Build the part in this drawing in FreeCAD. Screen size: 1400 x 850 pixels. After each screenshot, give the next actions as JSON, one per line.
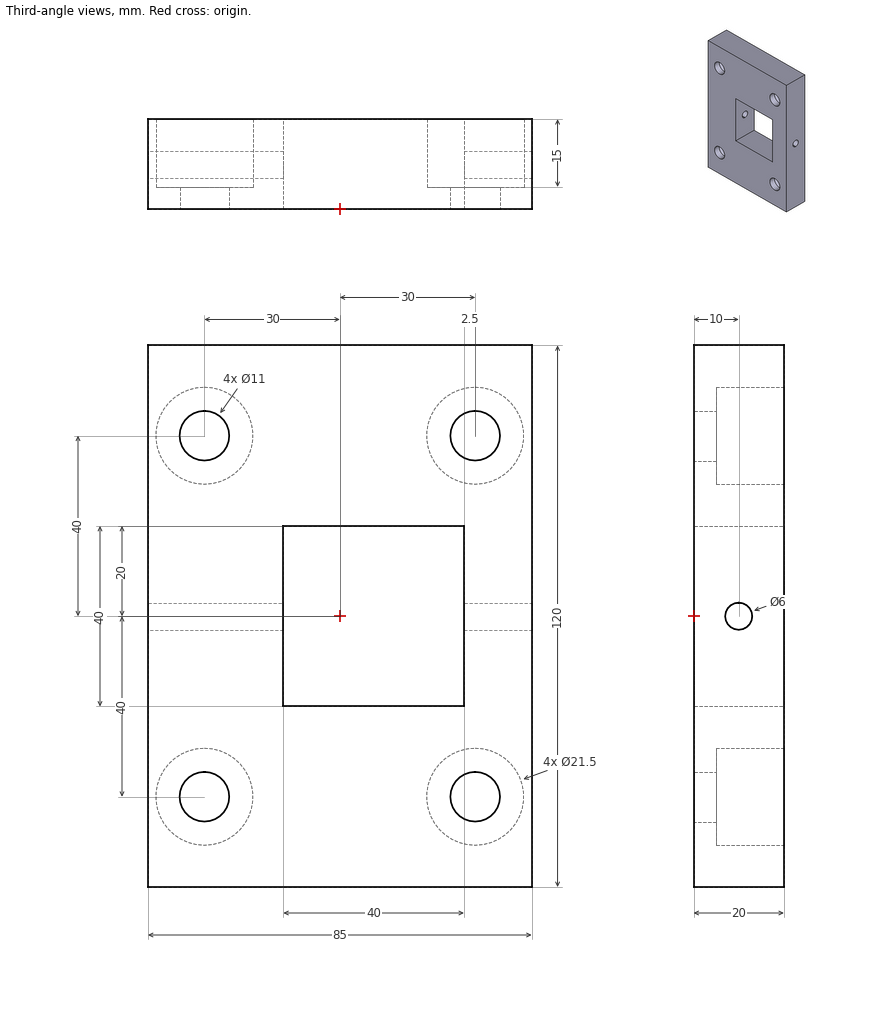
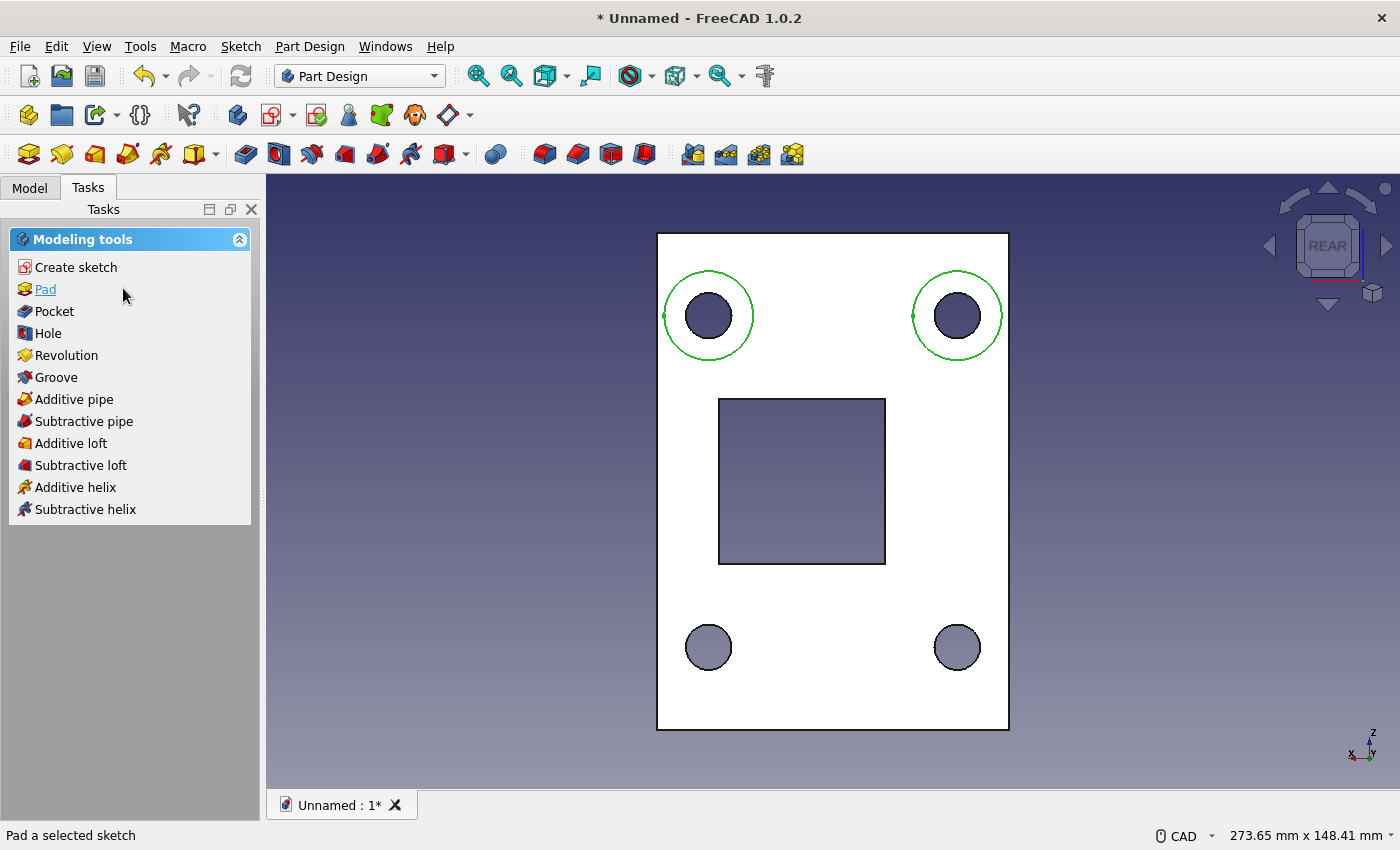
{"action": "left_click", "coordinate": [246, 154]}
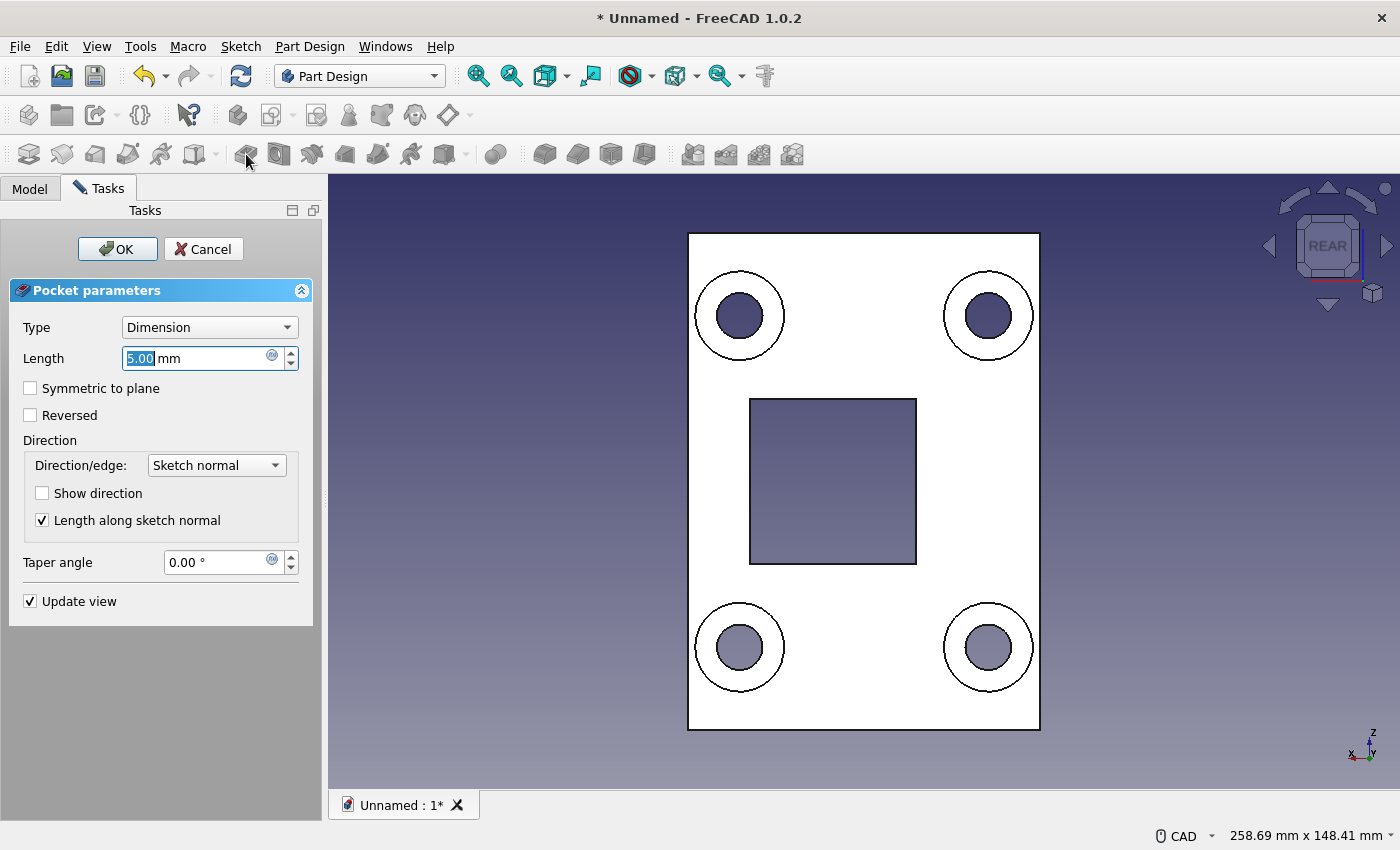
{"action": "type", "text": "15"}
{"action": "key", "text": "Tab"}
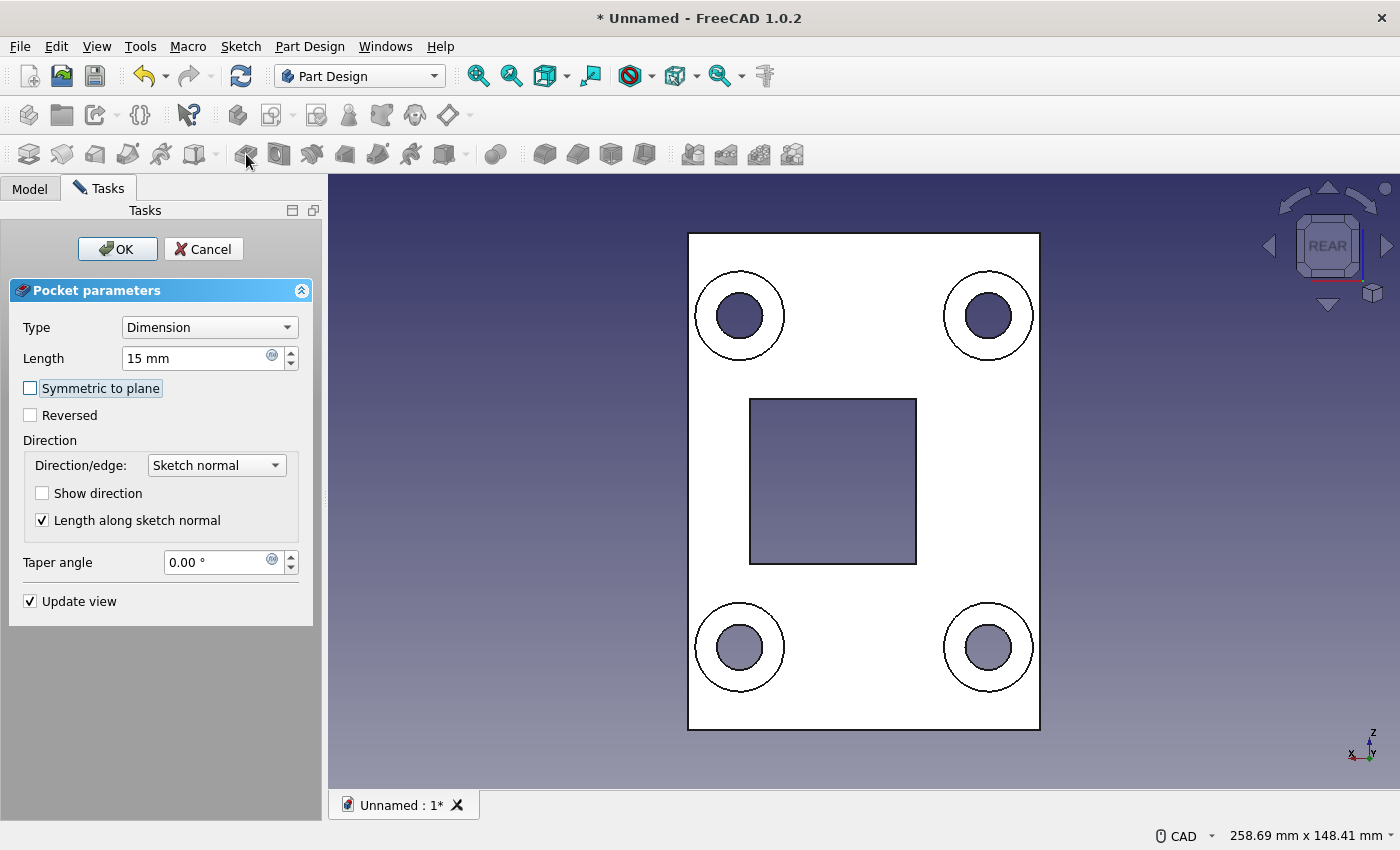
{"action": "left_click", "coordinate": [118, 249]}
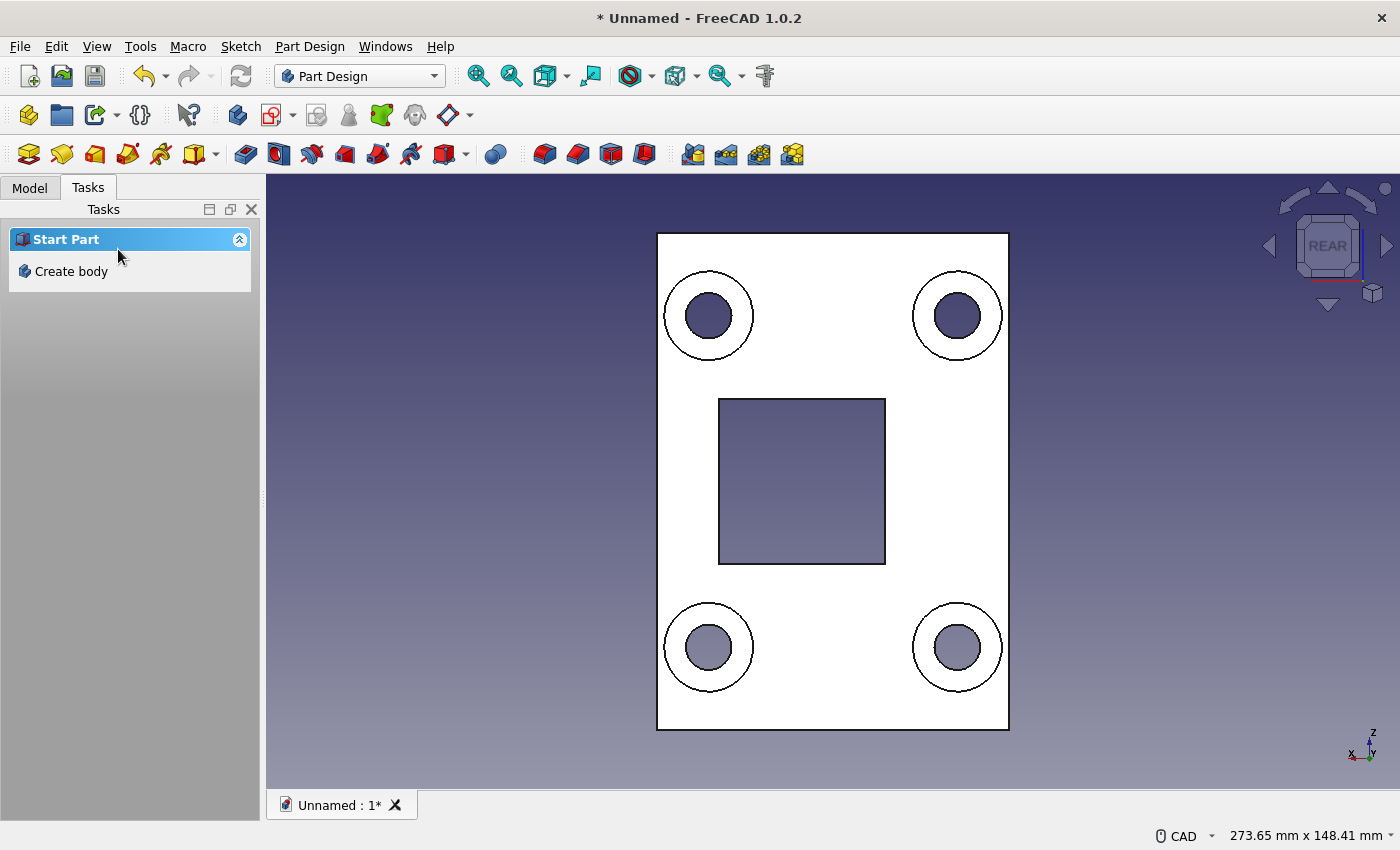
{"action": "key", "text": "6"}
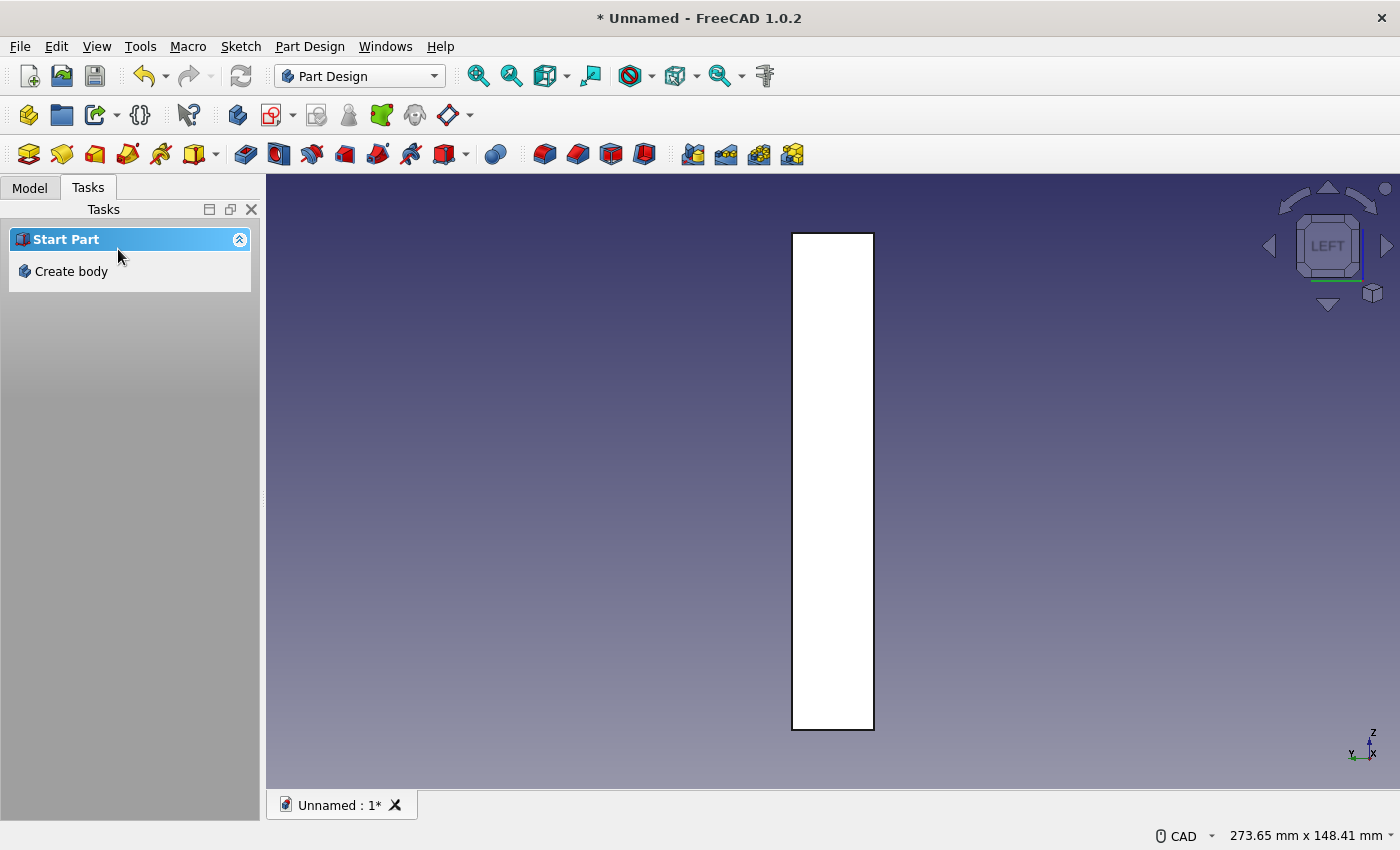
{"action": "left_click", "coordinate": [833, 481]}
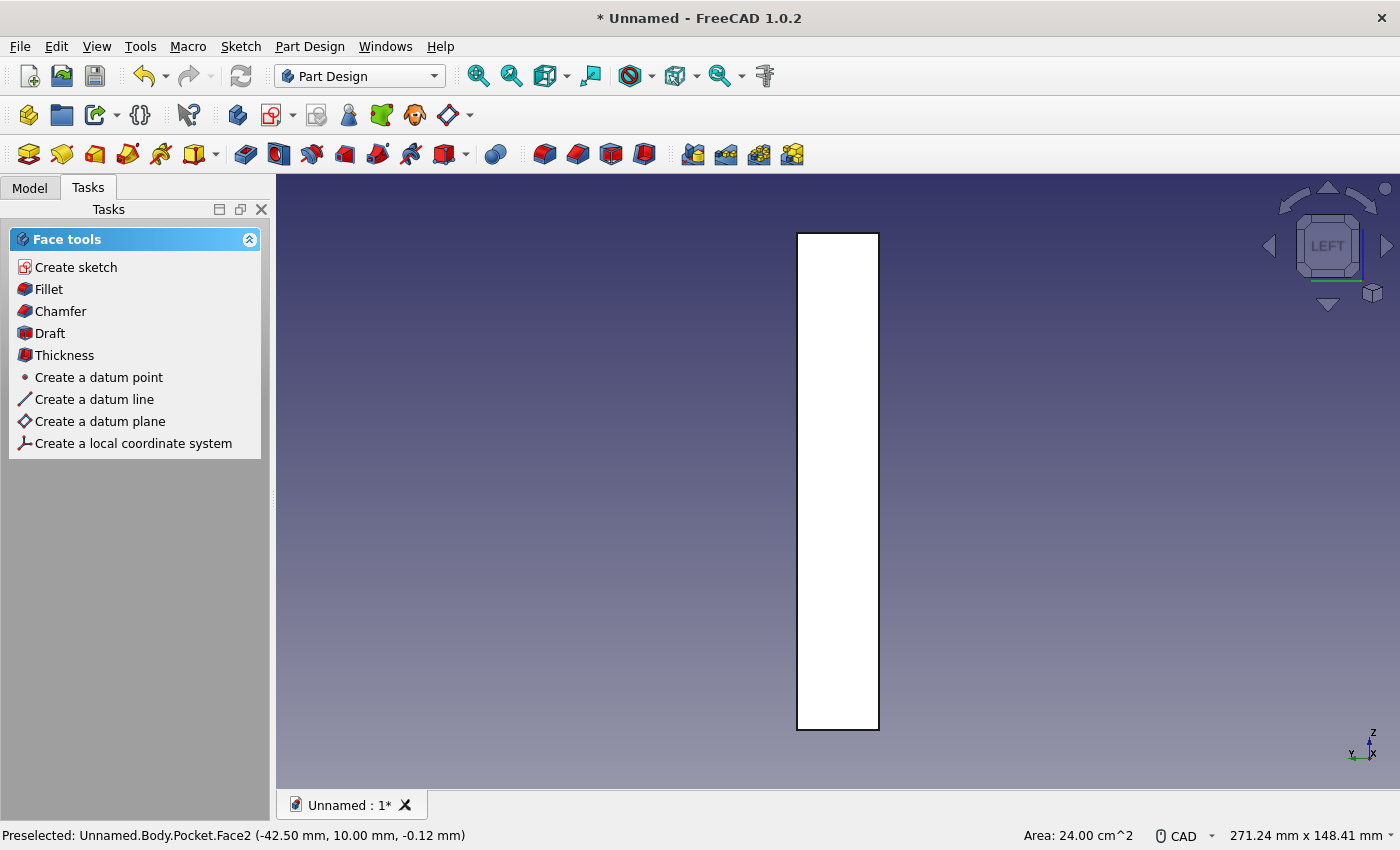
{"action": "left_click", "coordinate": [270, 116]}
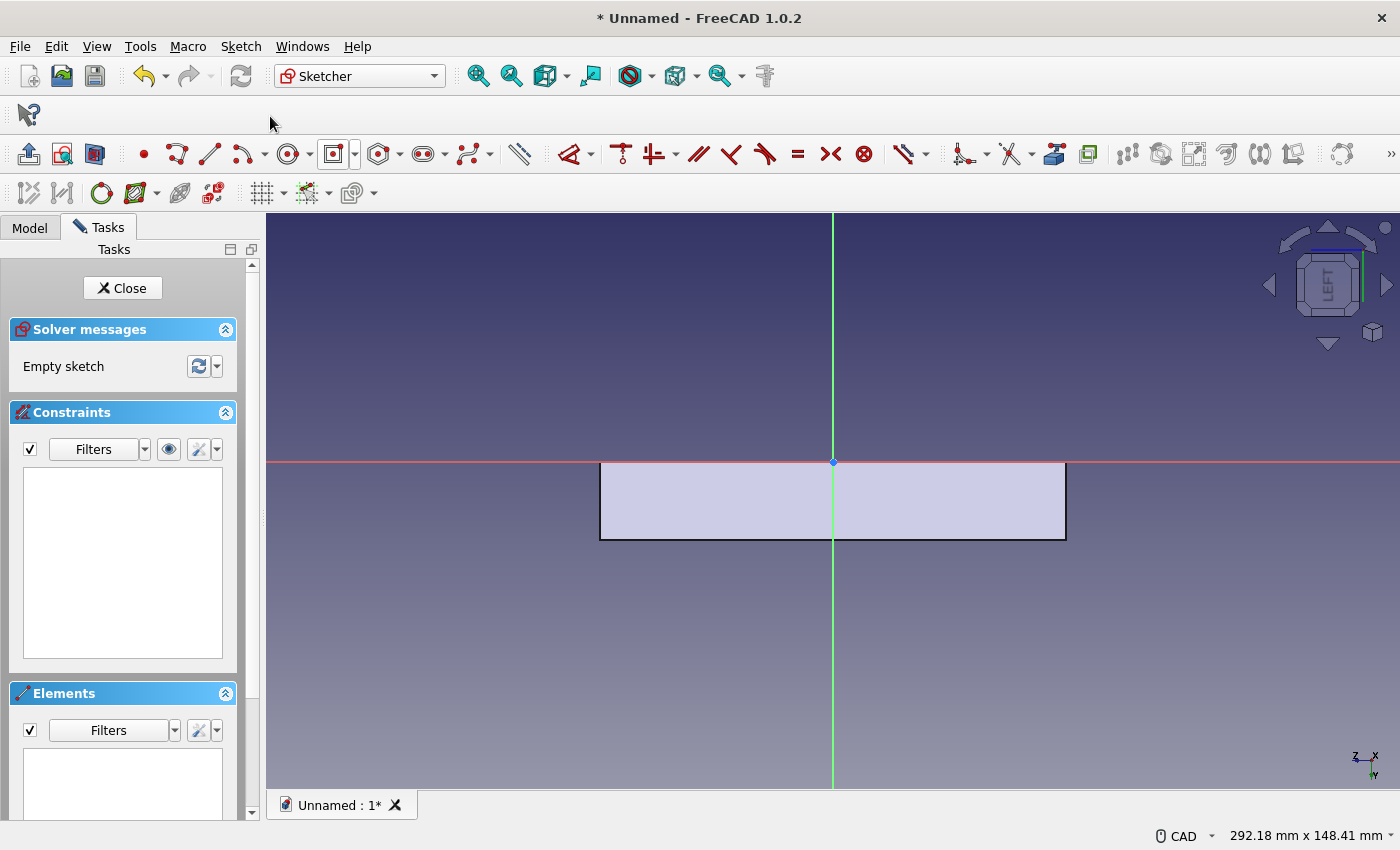
{"action": "scroll", "coordinate": [844, 485], "scroll_direction": "up", "scroll_amount": 10}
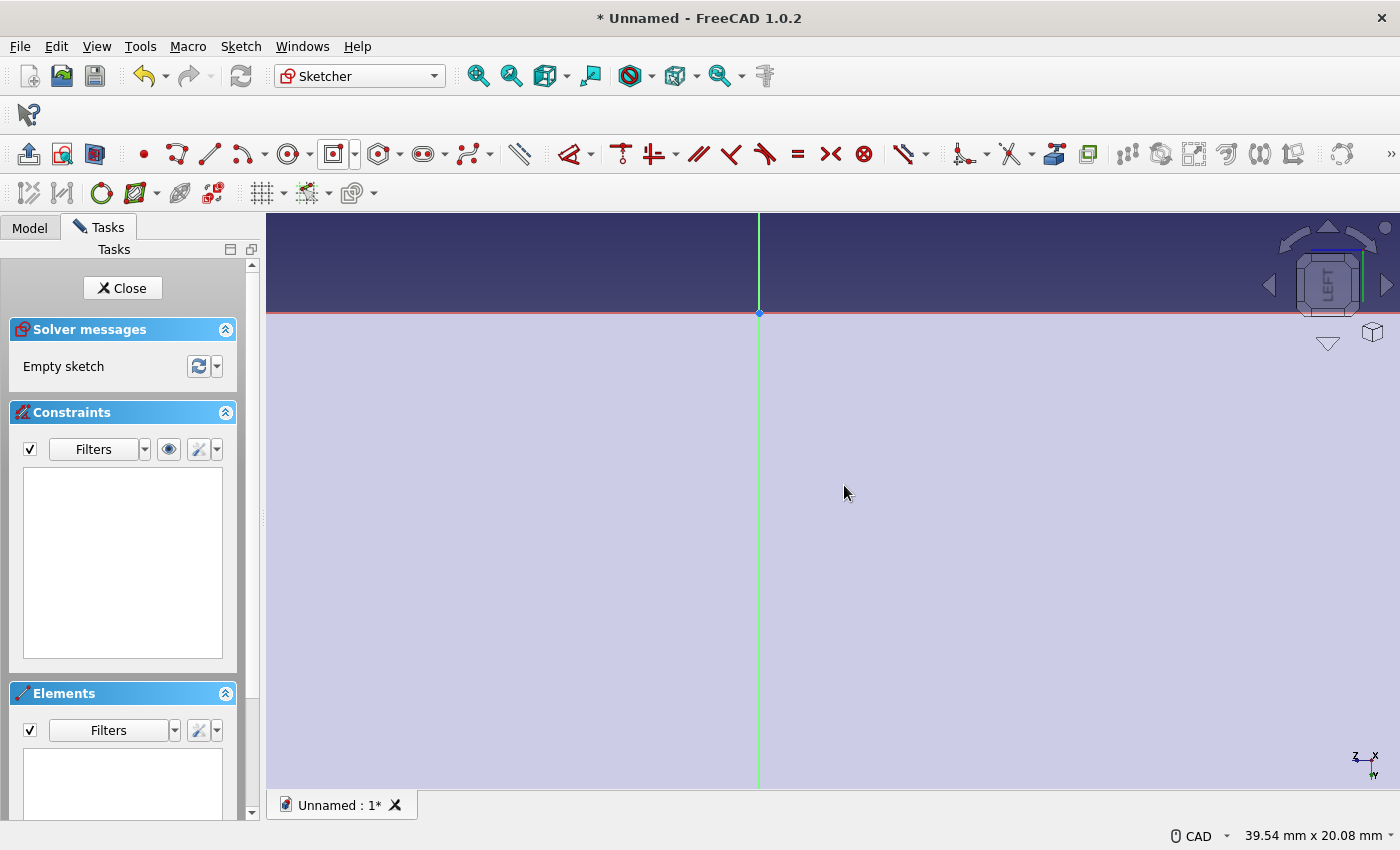
{"action": "key", "text": "g c"}